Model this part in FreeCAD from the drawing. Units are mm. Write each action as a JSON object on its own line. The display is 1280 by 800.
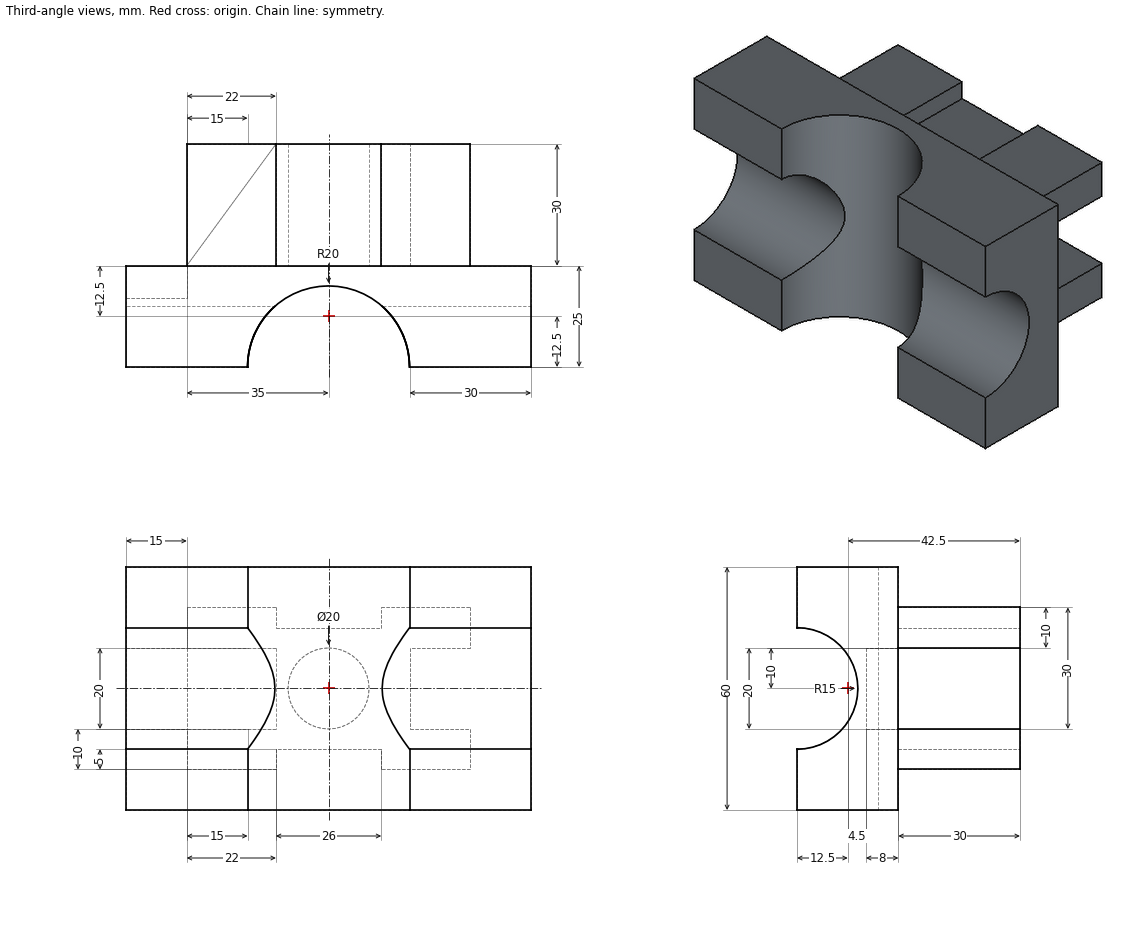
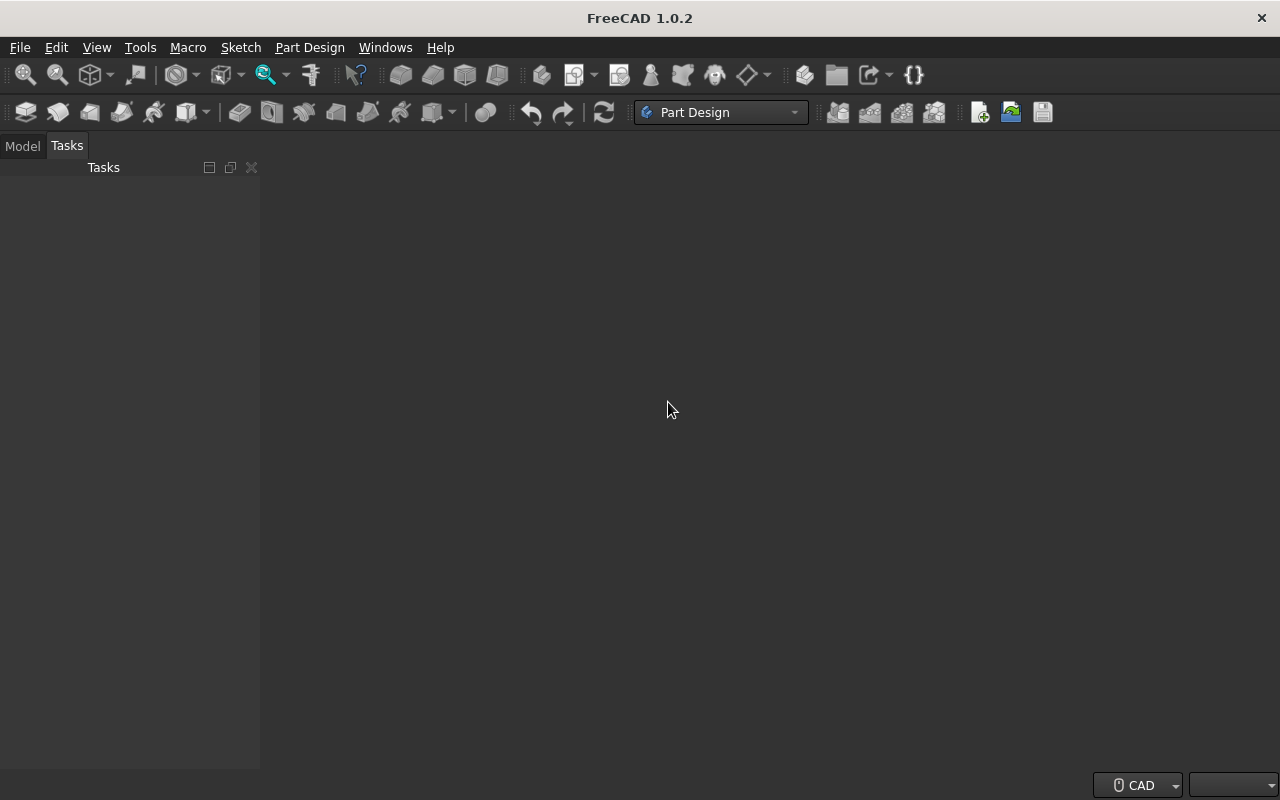
{"action": "left_click", "coordinate": [980, 112]}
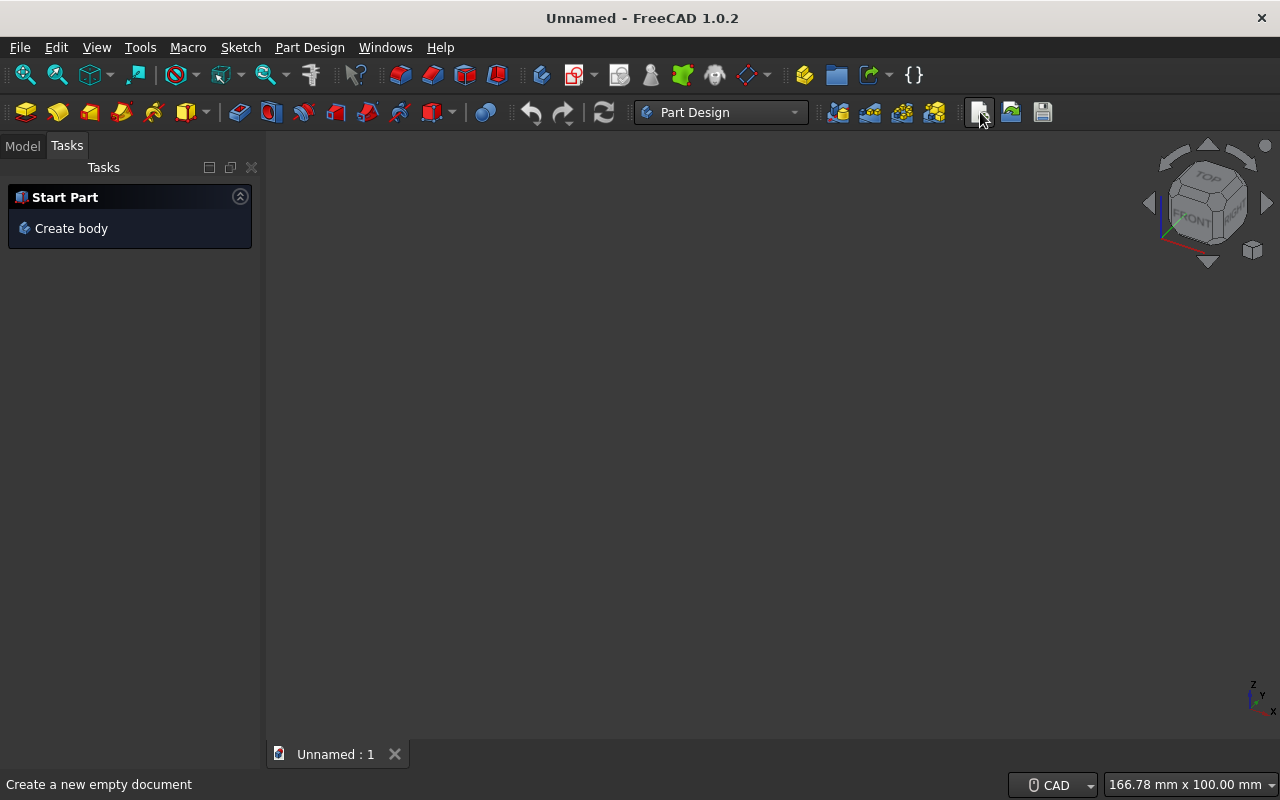
{"action": "left_click", "coordinate": [574, 76]}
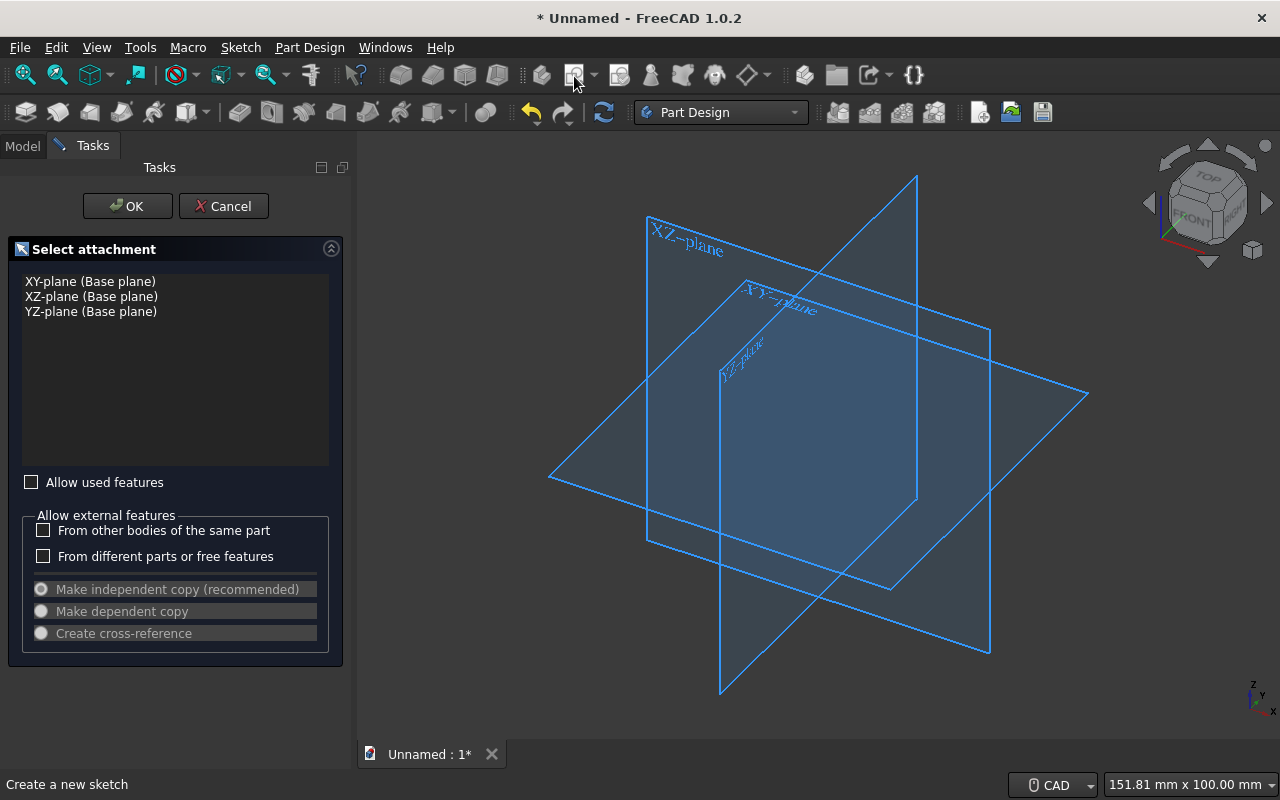
{"action": "left_click", "coordinate": [82, 282]}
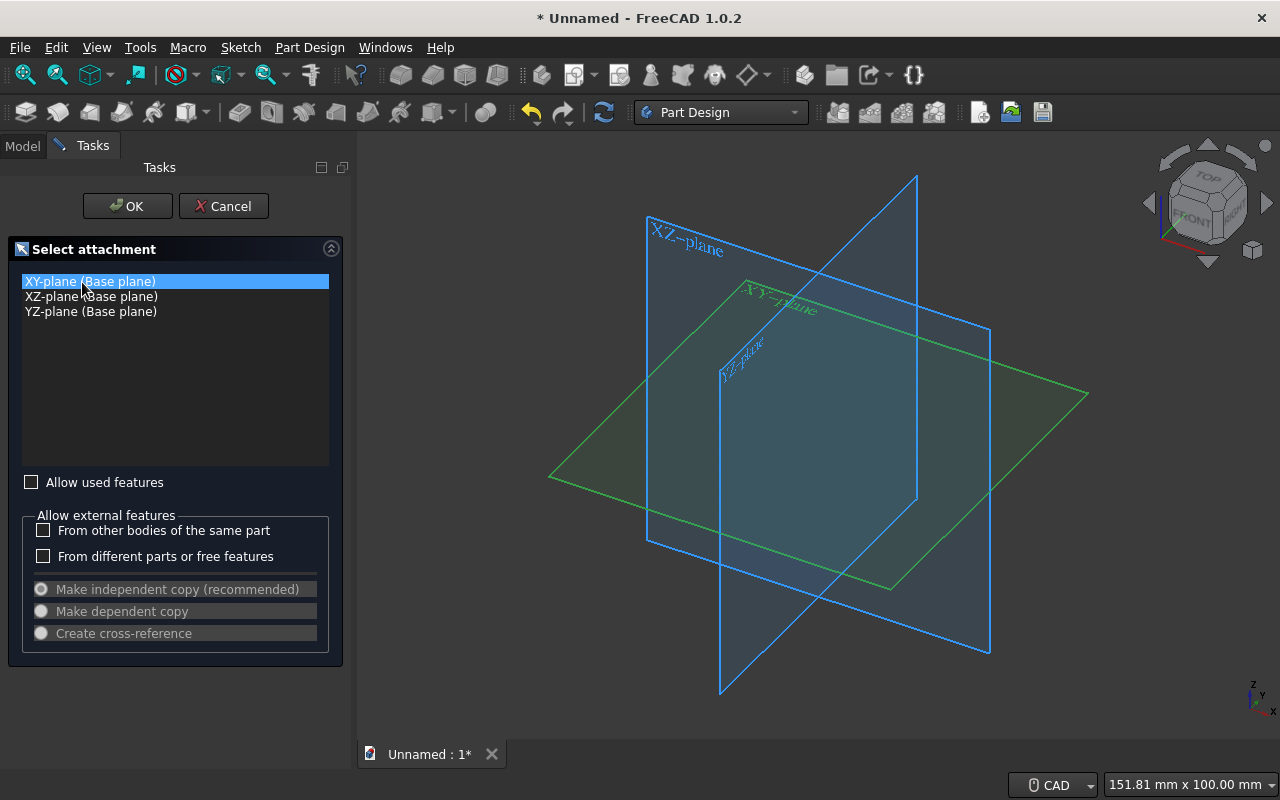
{"action": "left_click", "coordinate": [128, 206]}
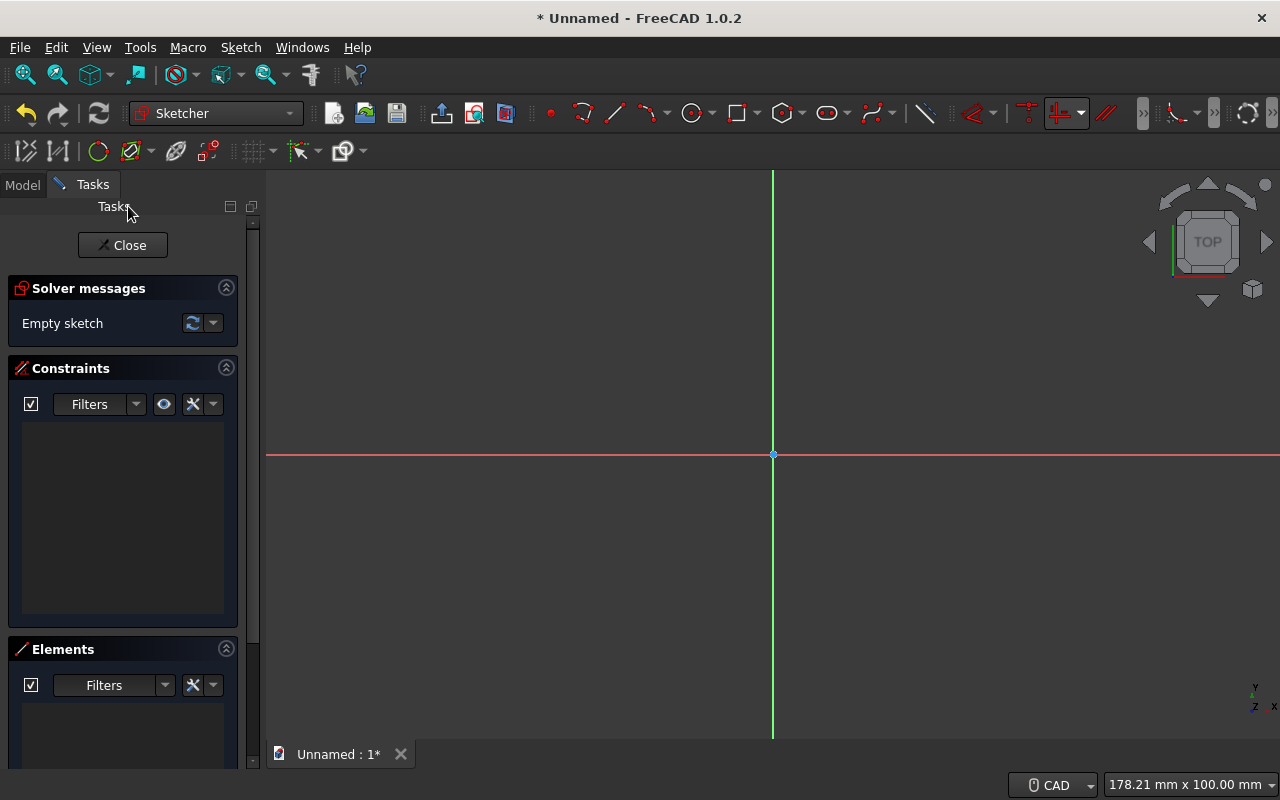
{"action": "left_click", "coordinate": [584, 114]}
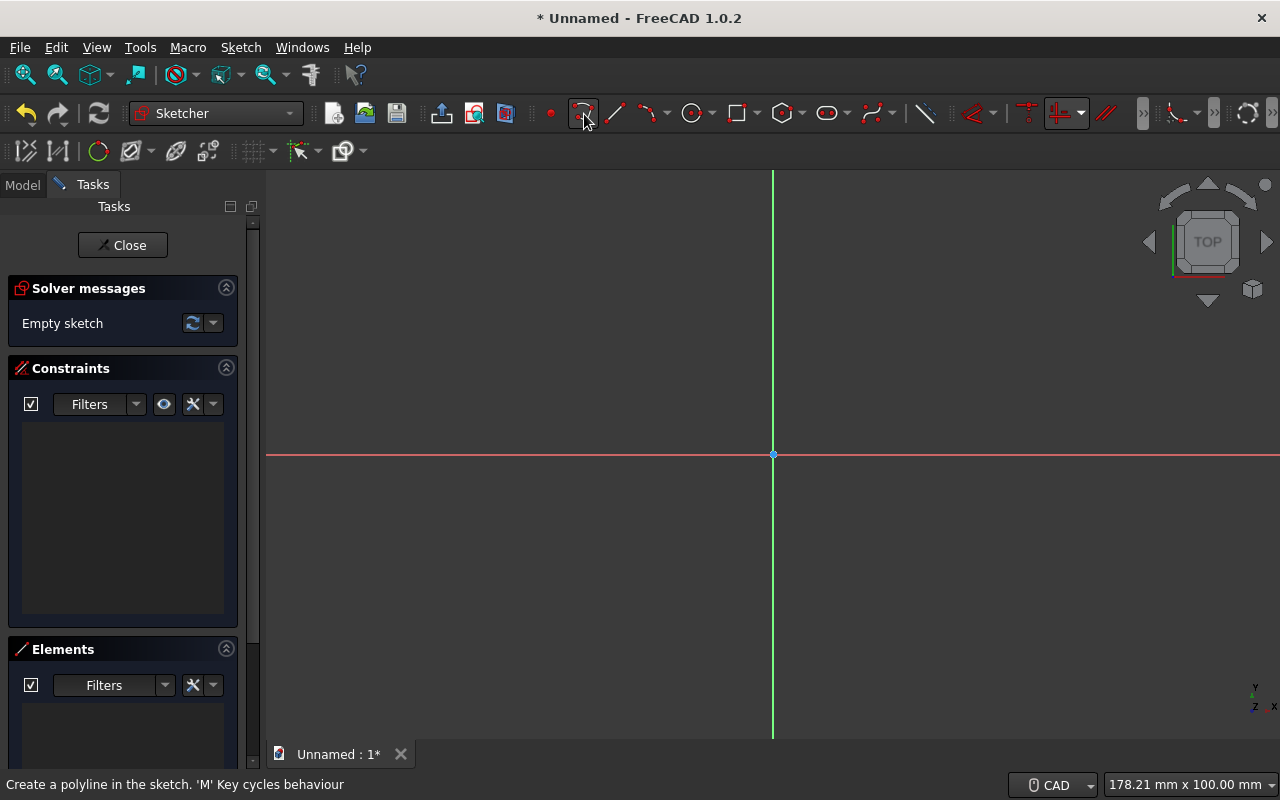
{"action": "left_click", "coordinate": [887, 526]}
{"action": "left_click", "coordinate": [1058, 526]}
{"action": "left_click", "coordinate": [1058, 383]}
{"action": "left_click", "coordinate": [488, 383]}
{"action": "left_click", "coordinate": [488, 526]}
{"action": "left_click", "coordinate": [659, 526]}
{"action": "right_click", "coordinate": [659, 526]}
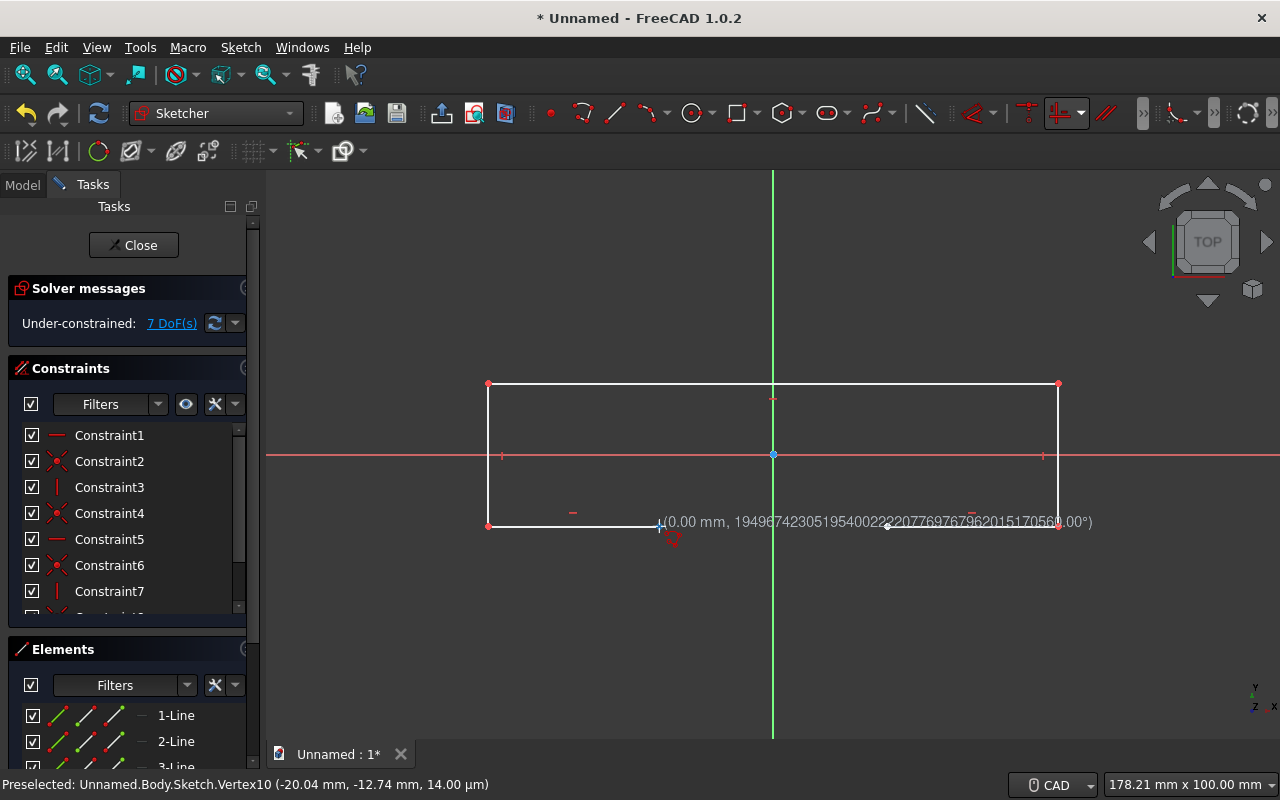
{"action": "left_click", "coordinate": [648, 114]}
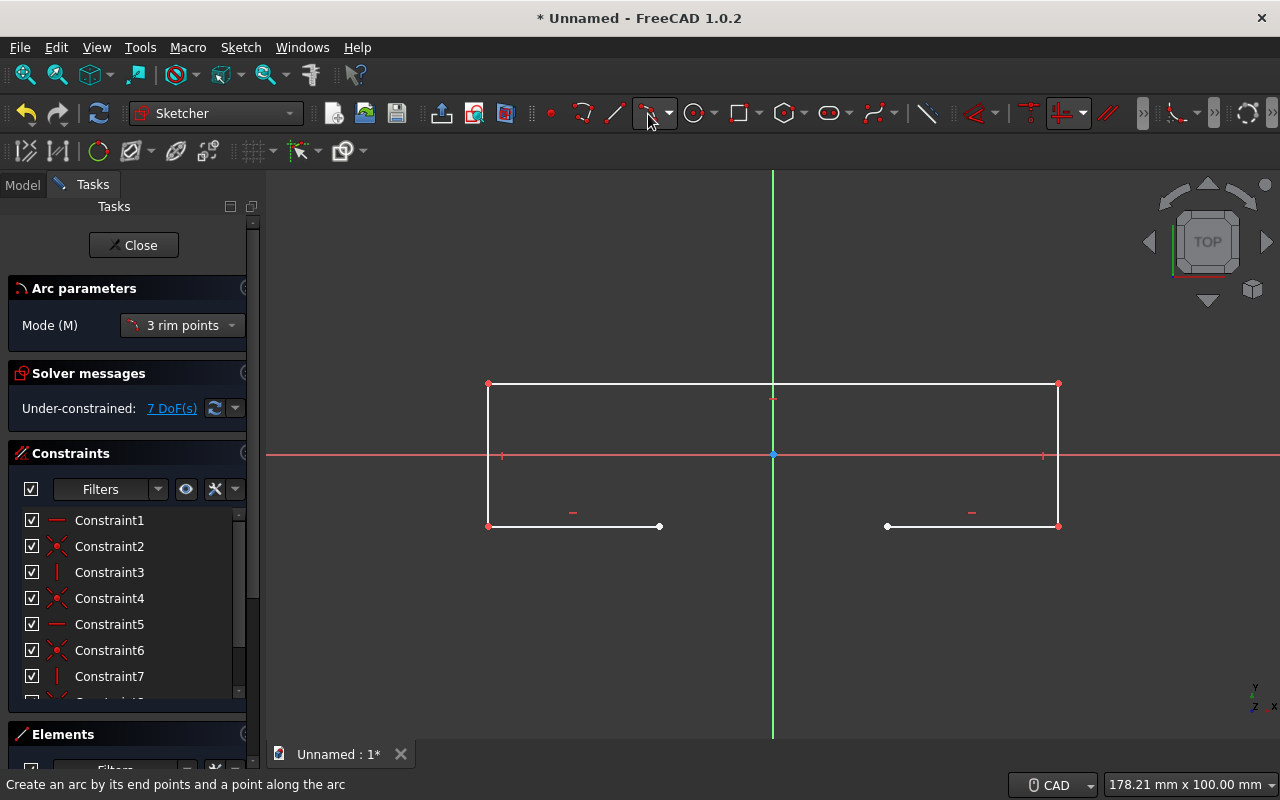
{"action": "left_click", "coordinate": [659, 527]}
{"action": "left_click", "coordinate": [887, 527]}
{"action": "left_click", "coordinate": [808, 417]}
{"action": "key", "text": "Escape"}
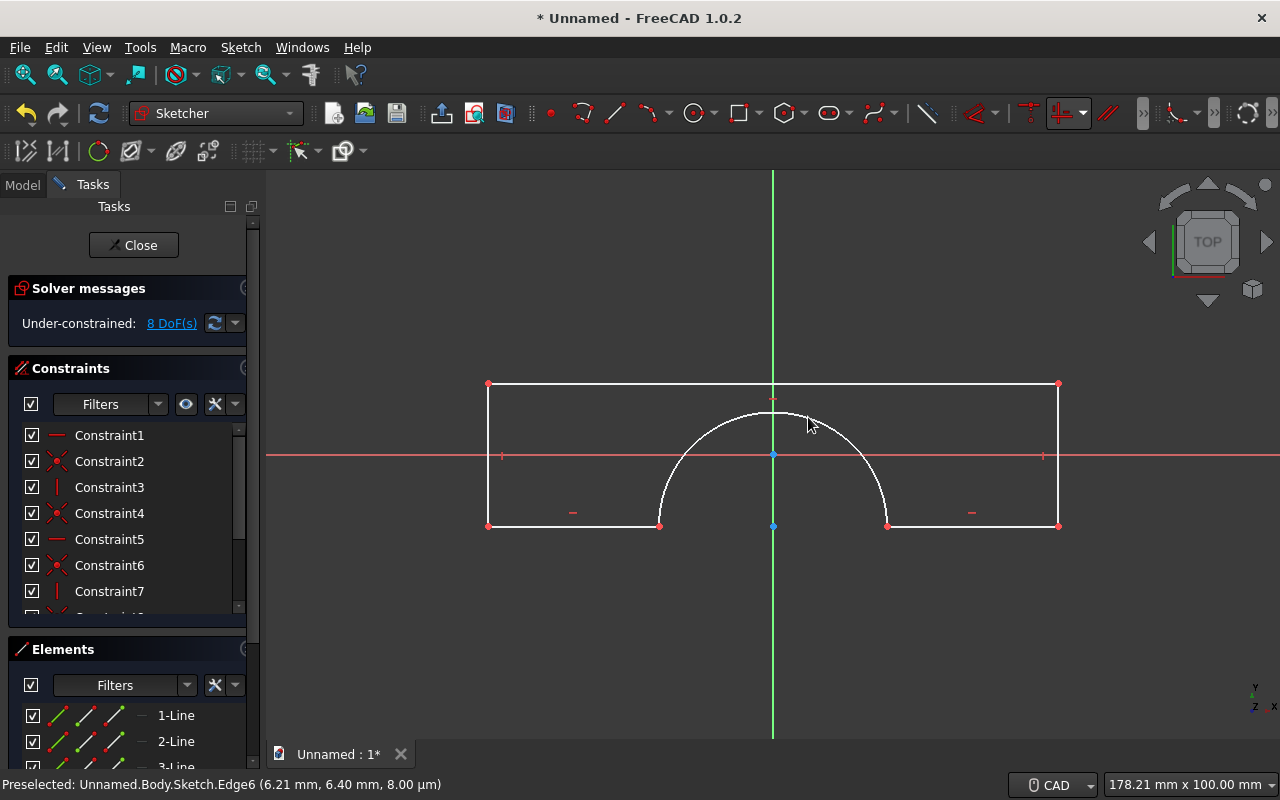
{"action": "left_click", "coordinate": [773, 526]}